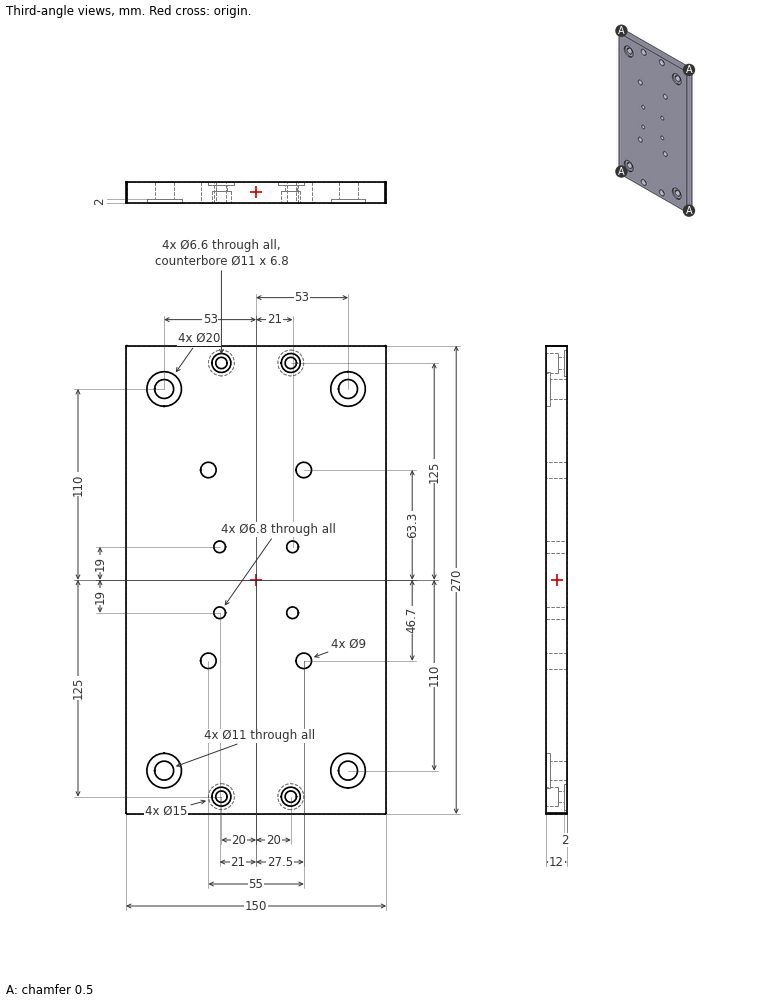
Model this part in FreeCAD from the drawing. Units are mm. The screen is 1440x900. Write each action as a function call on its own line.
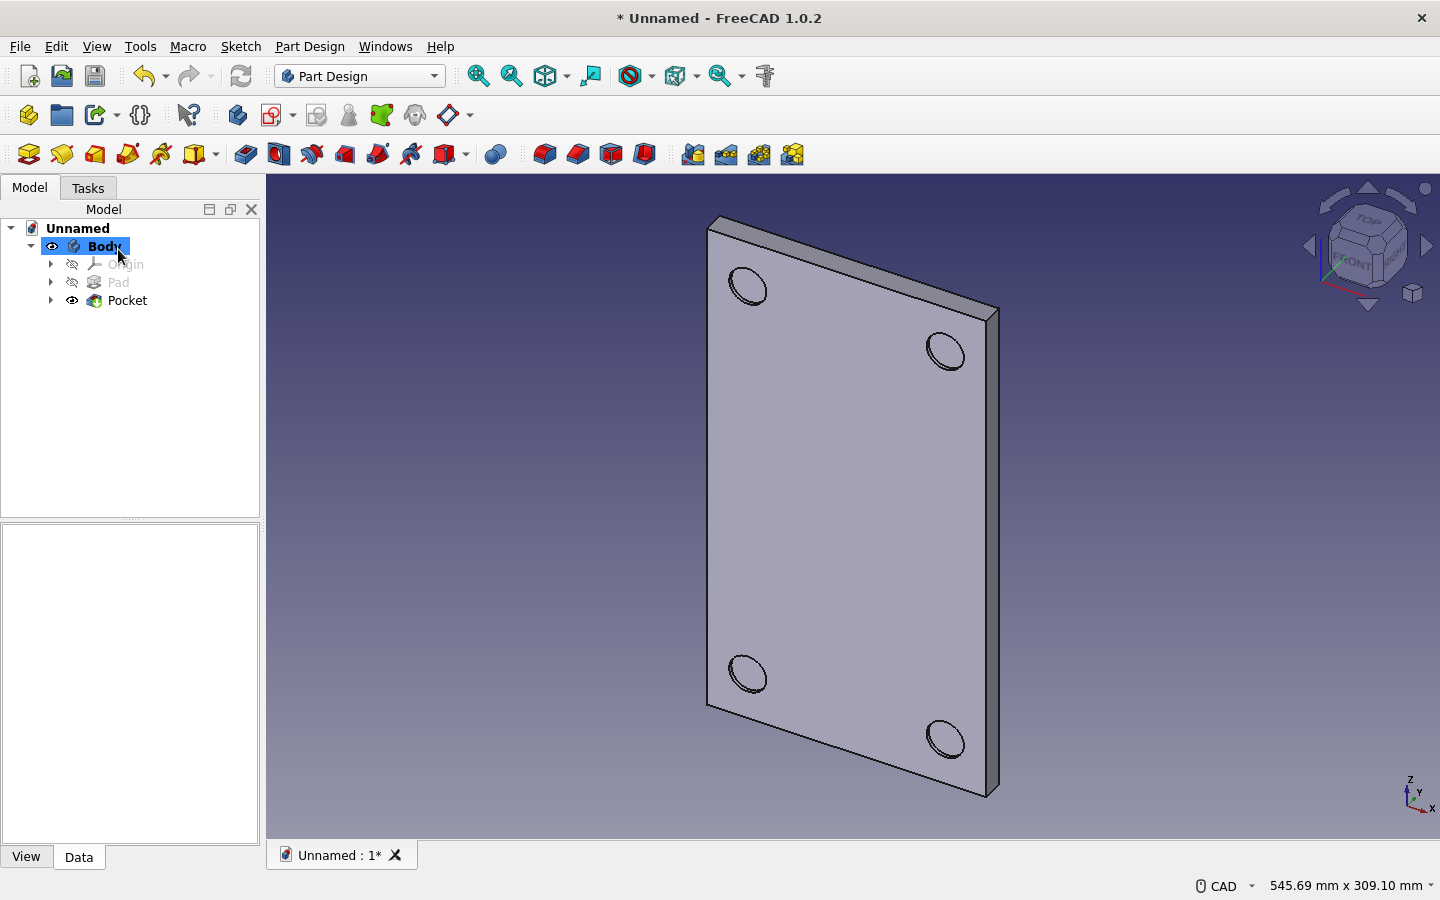
key(4)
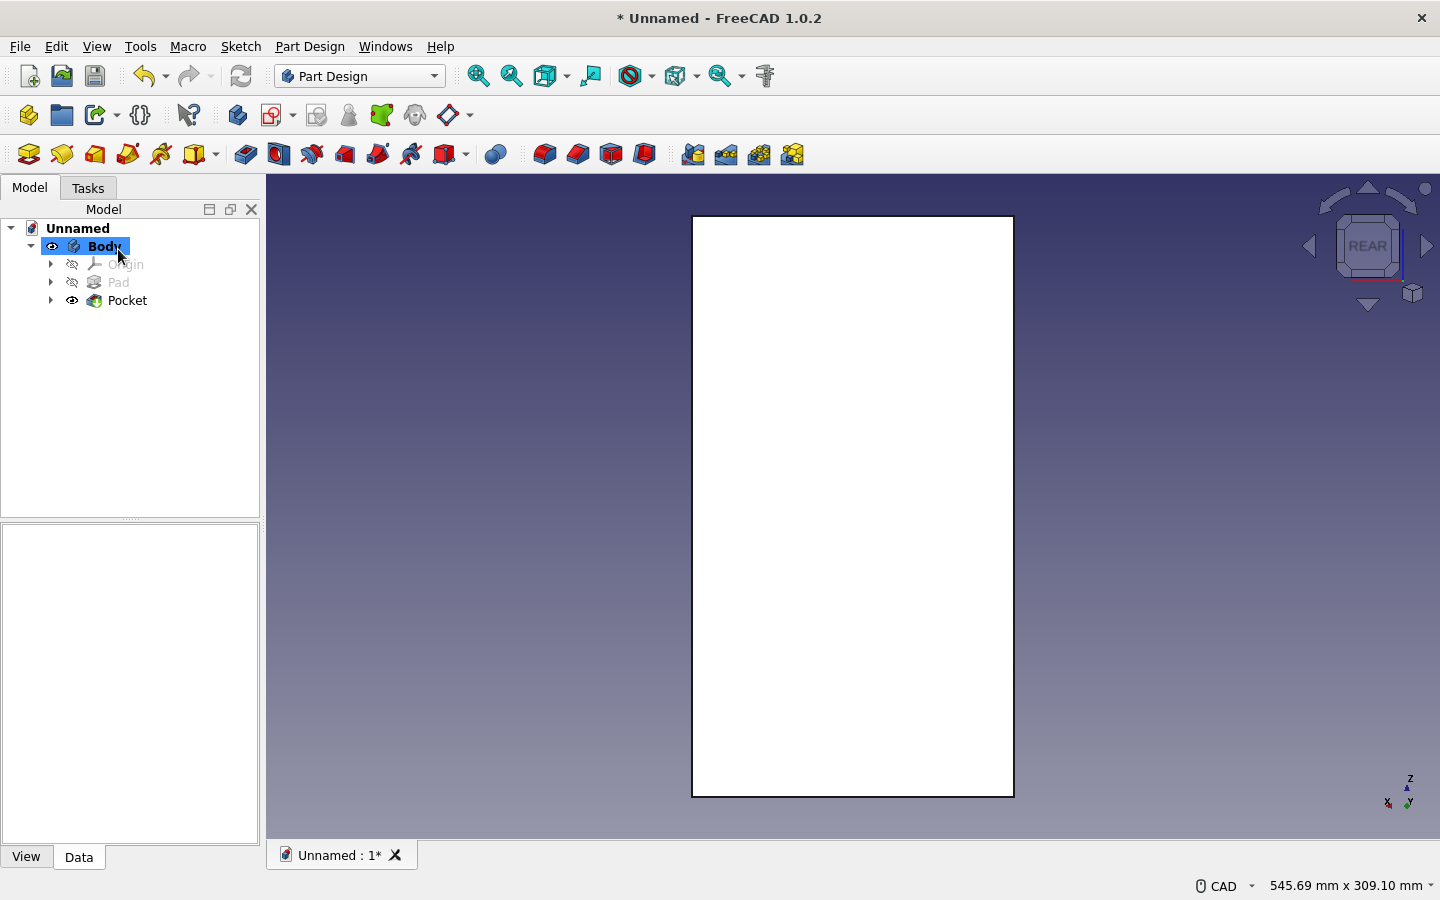
click(853, 423)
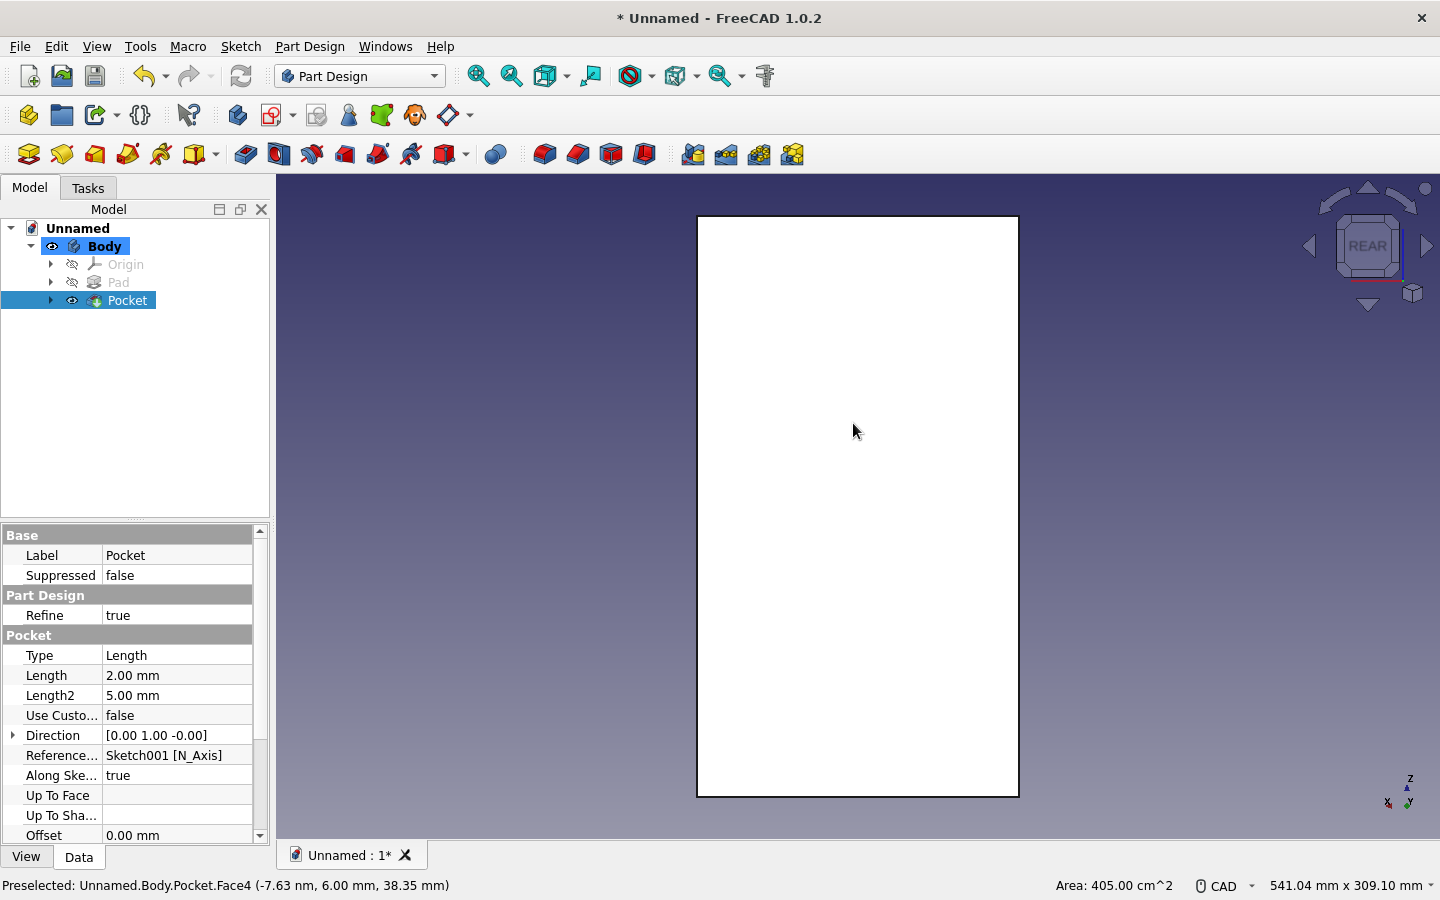
click(270, 116)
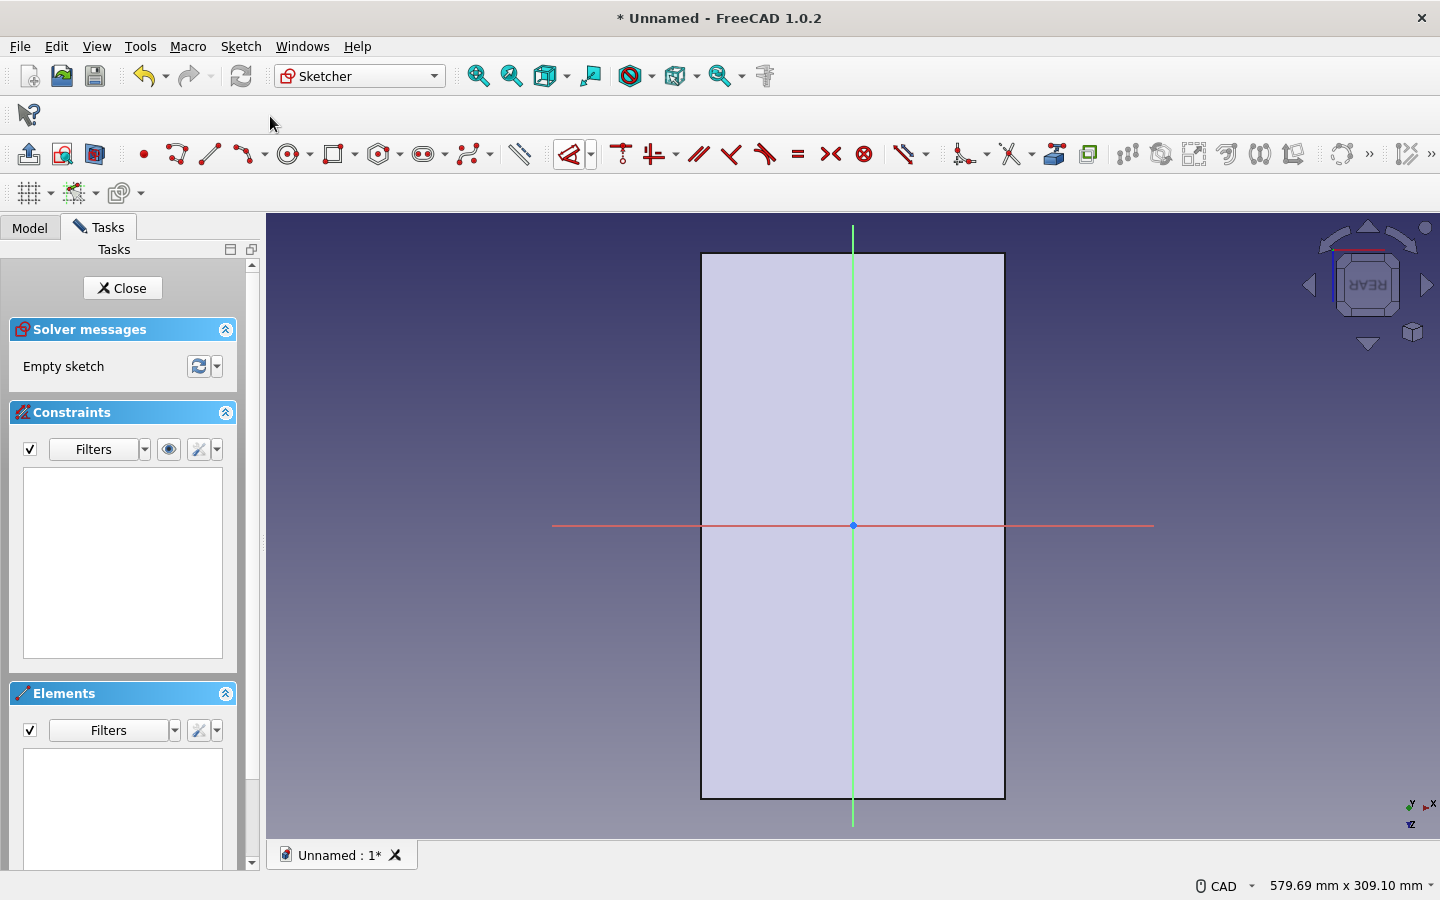
key(g)
key(c)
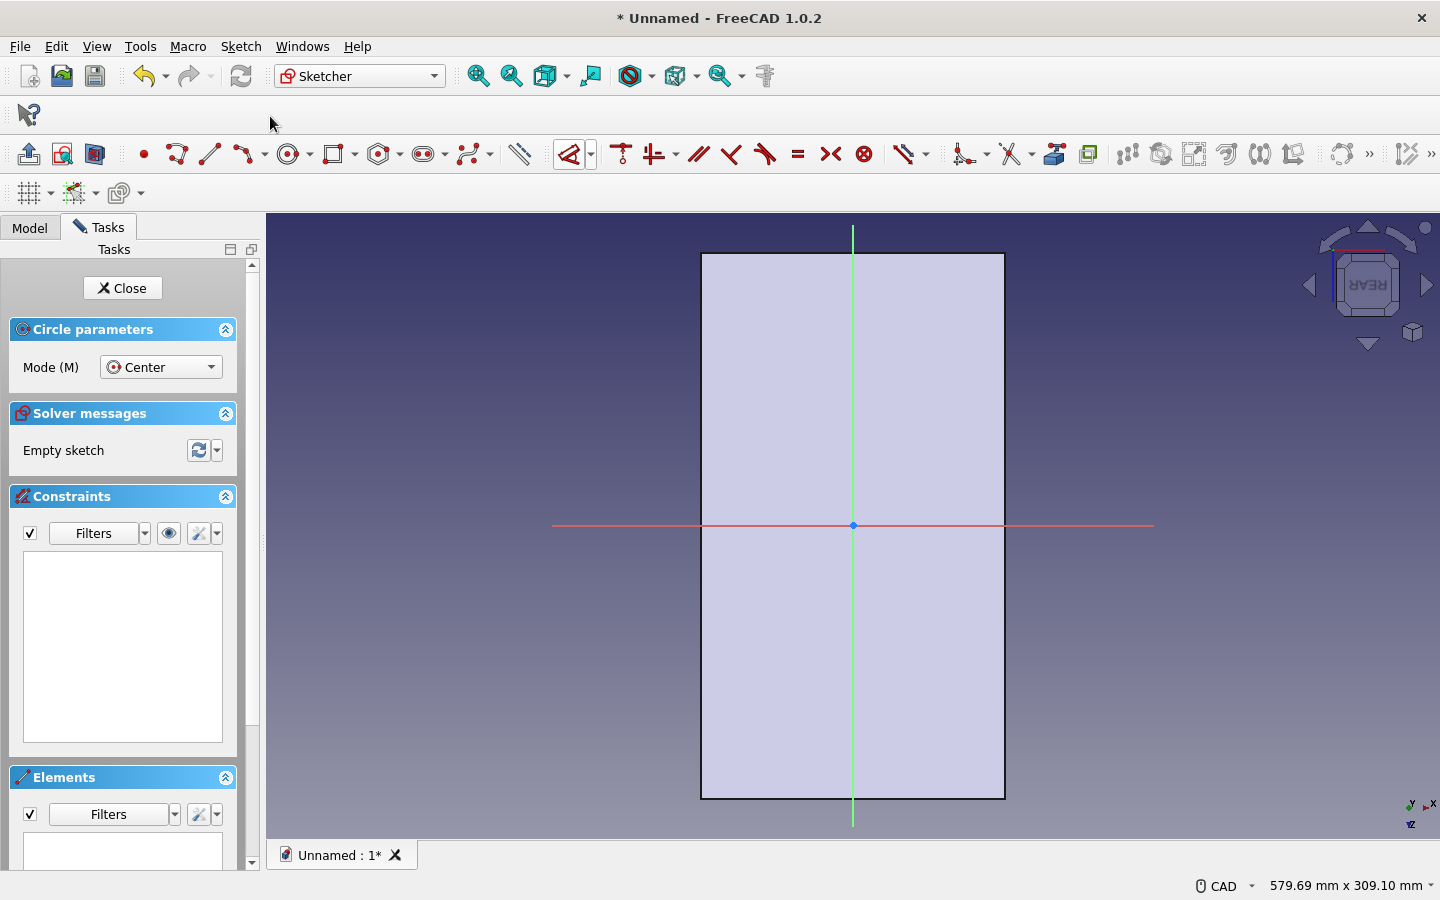
scroll(746, 303, up, 4)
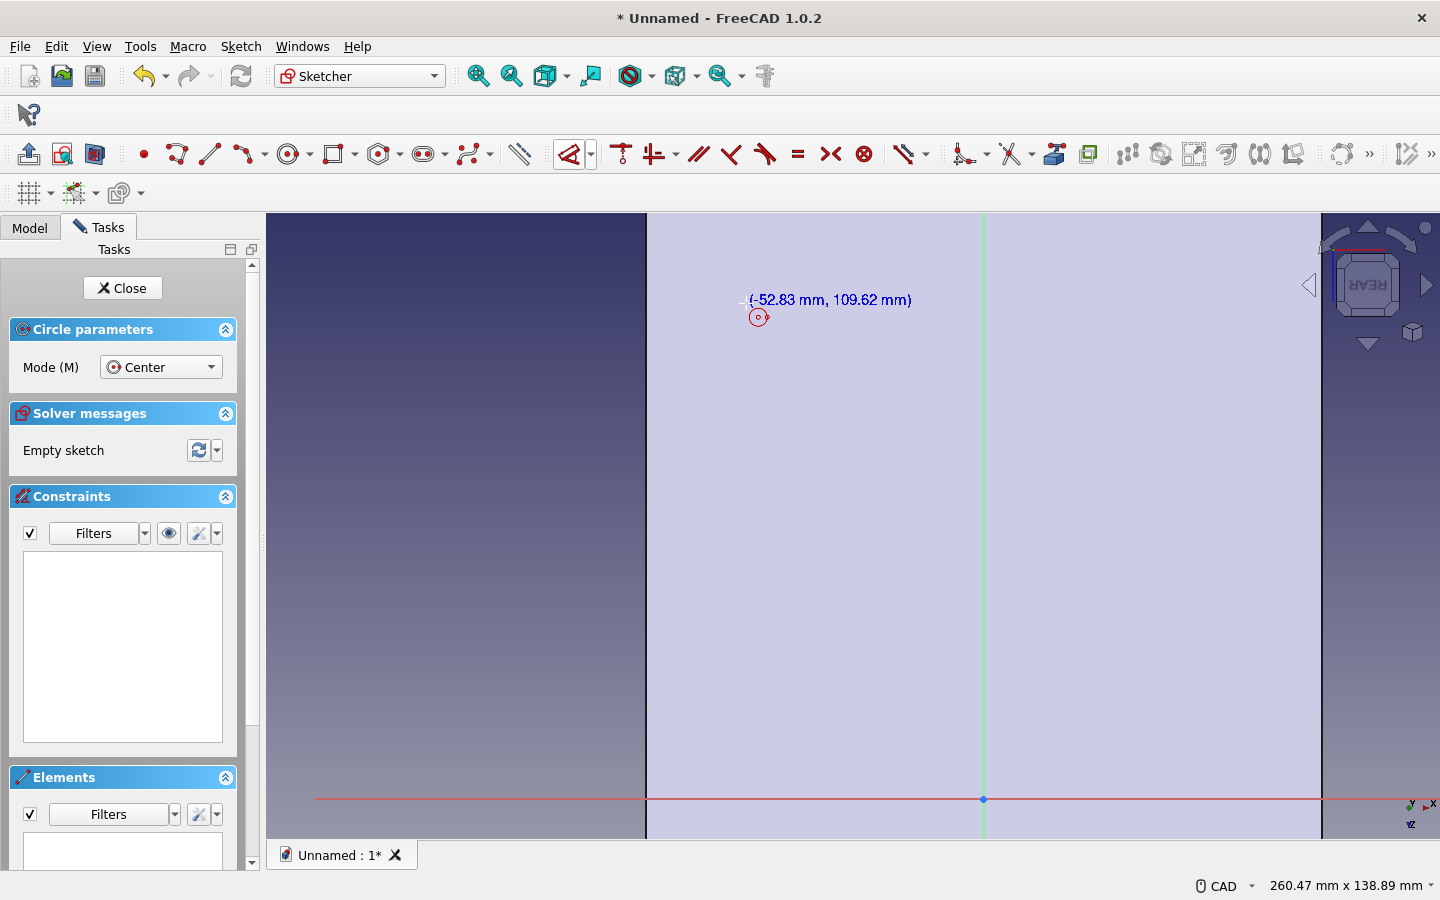
click(745, 303)
click(762, 286)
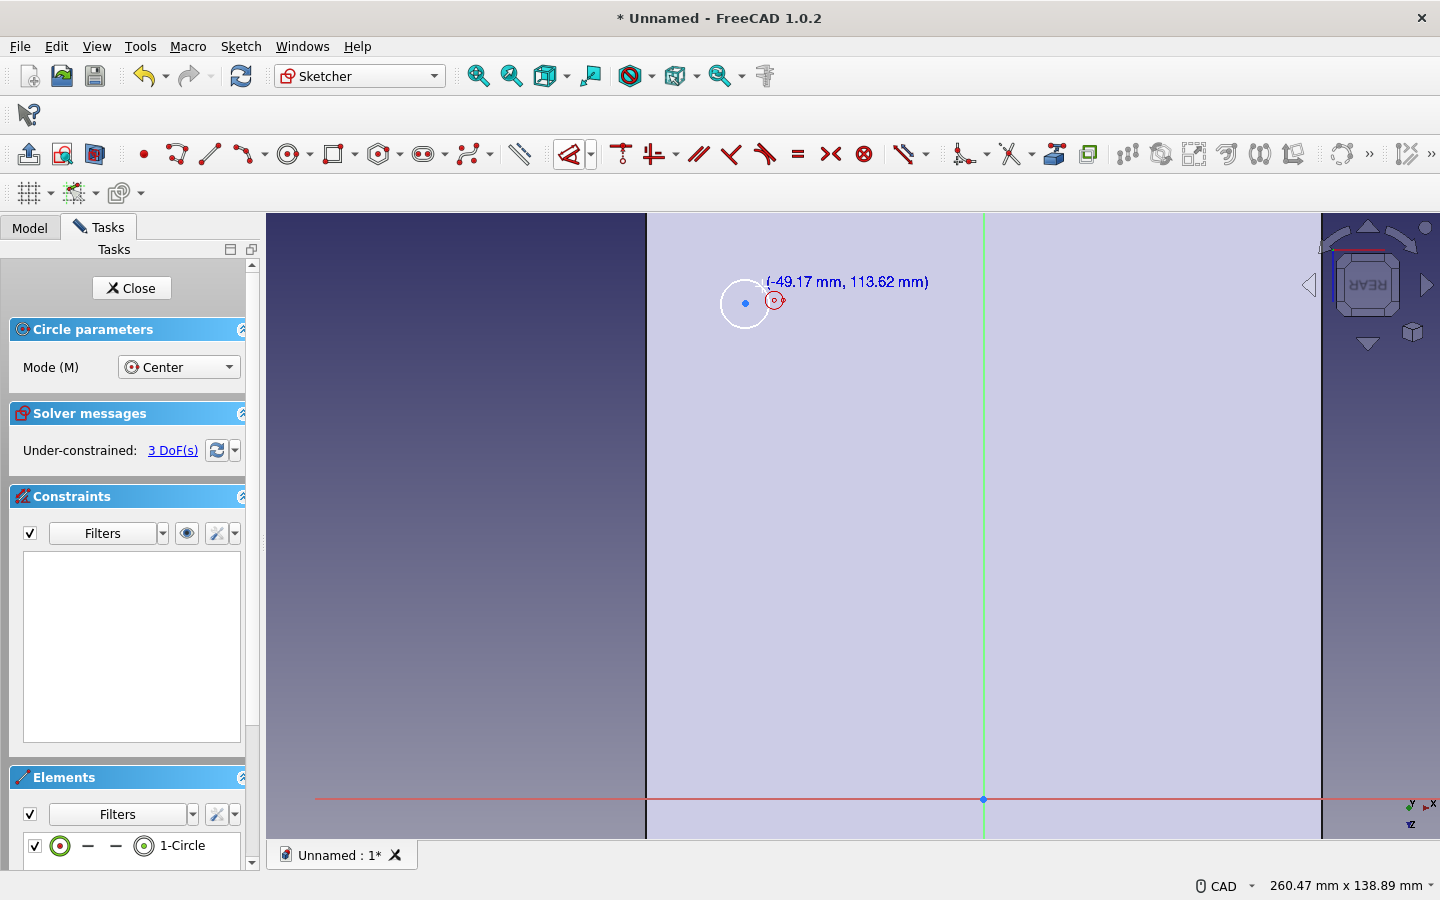
click(1223, 303)
click(1240, 286)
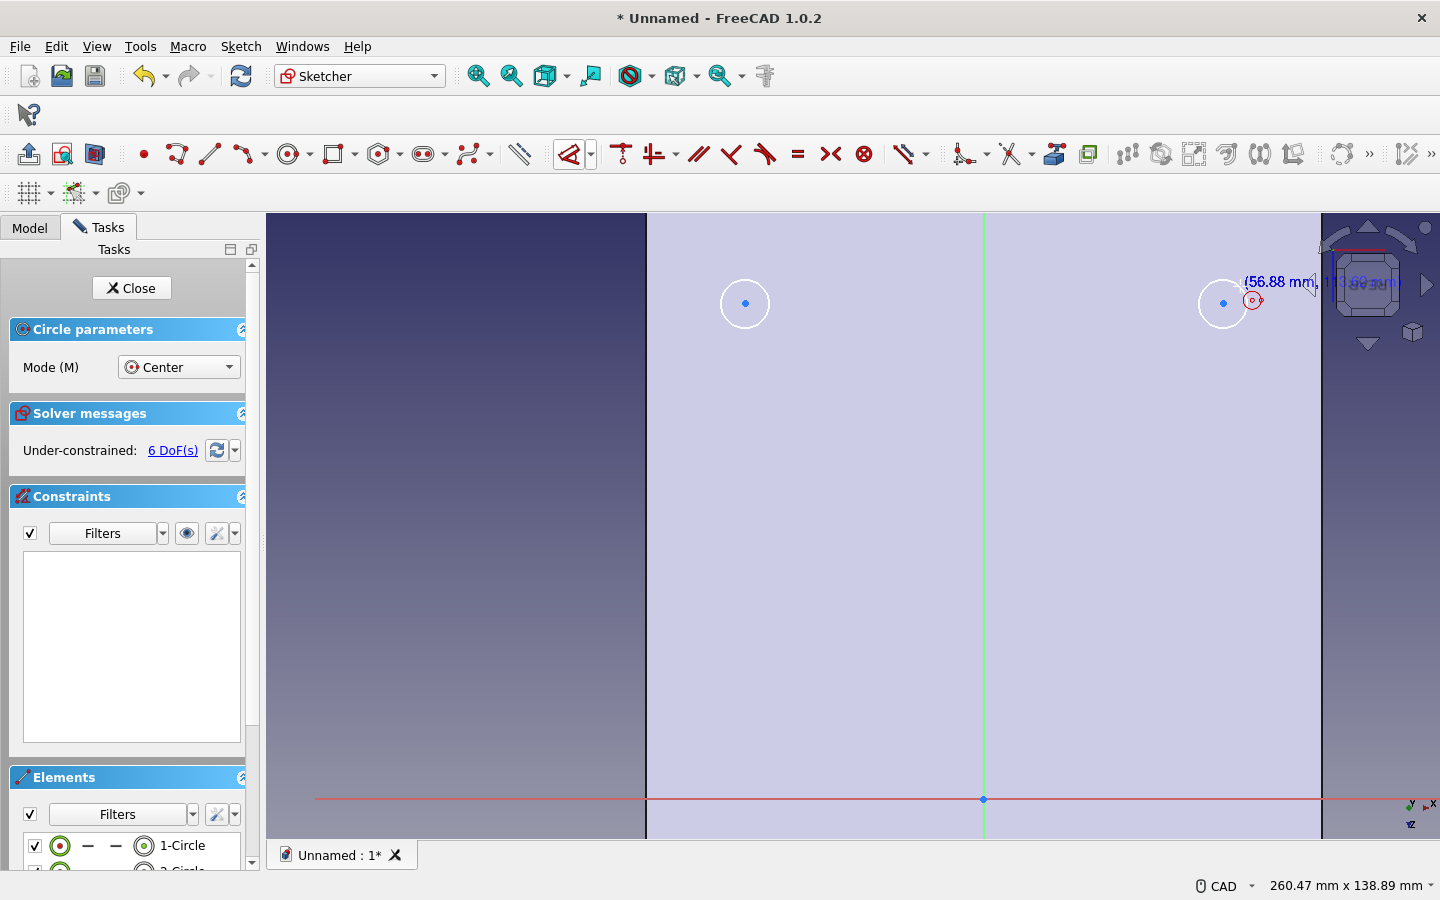
scroll(669, 367, down, 5)